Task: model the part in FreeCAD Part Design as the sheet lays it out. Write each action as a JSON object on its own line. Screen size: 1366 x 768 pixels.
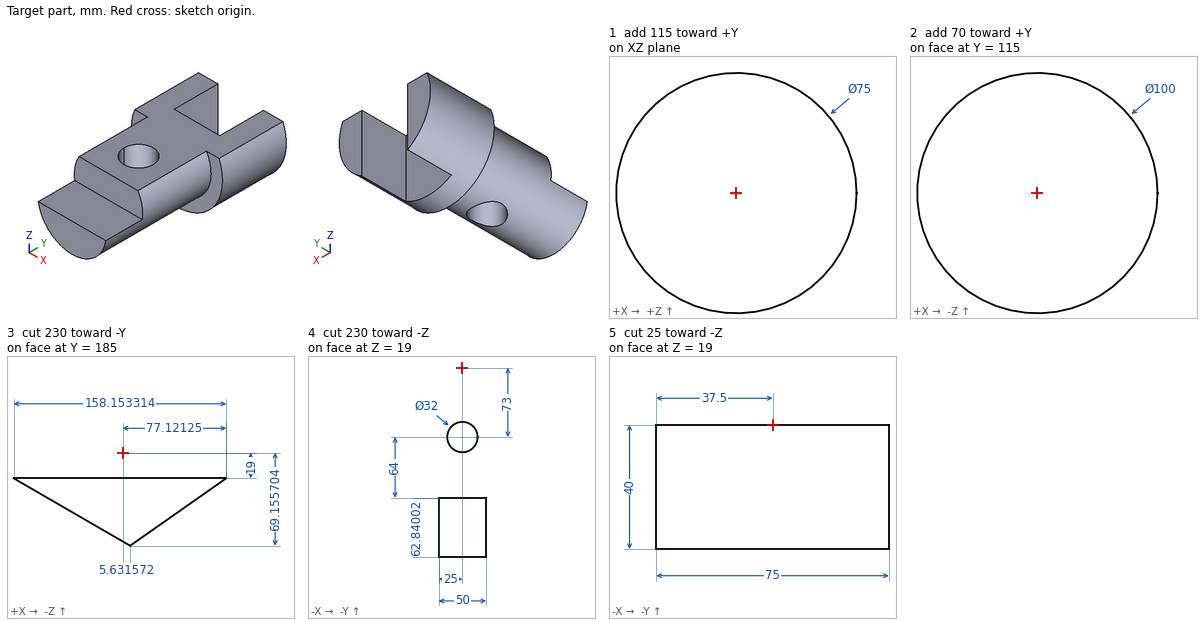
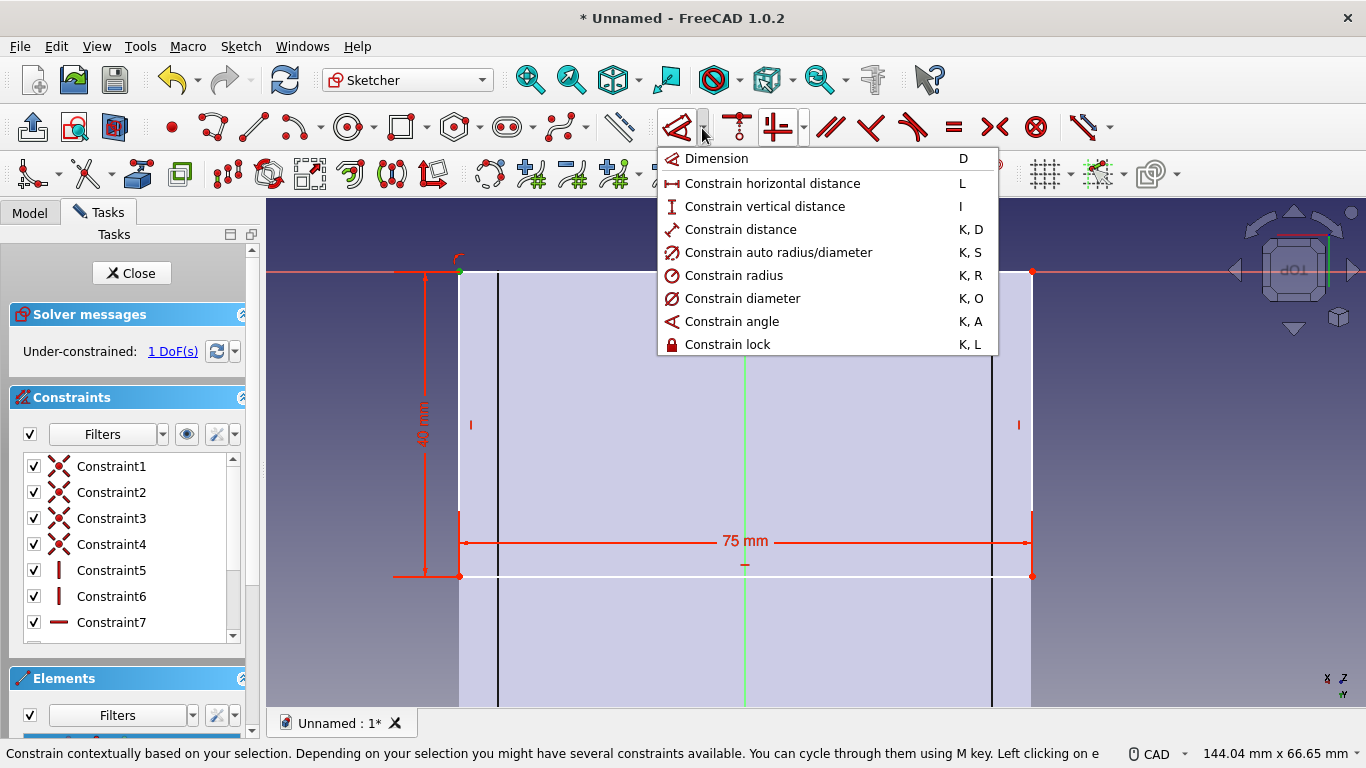
{"action": "left_click", "coordinate": [828, 184]}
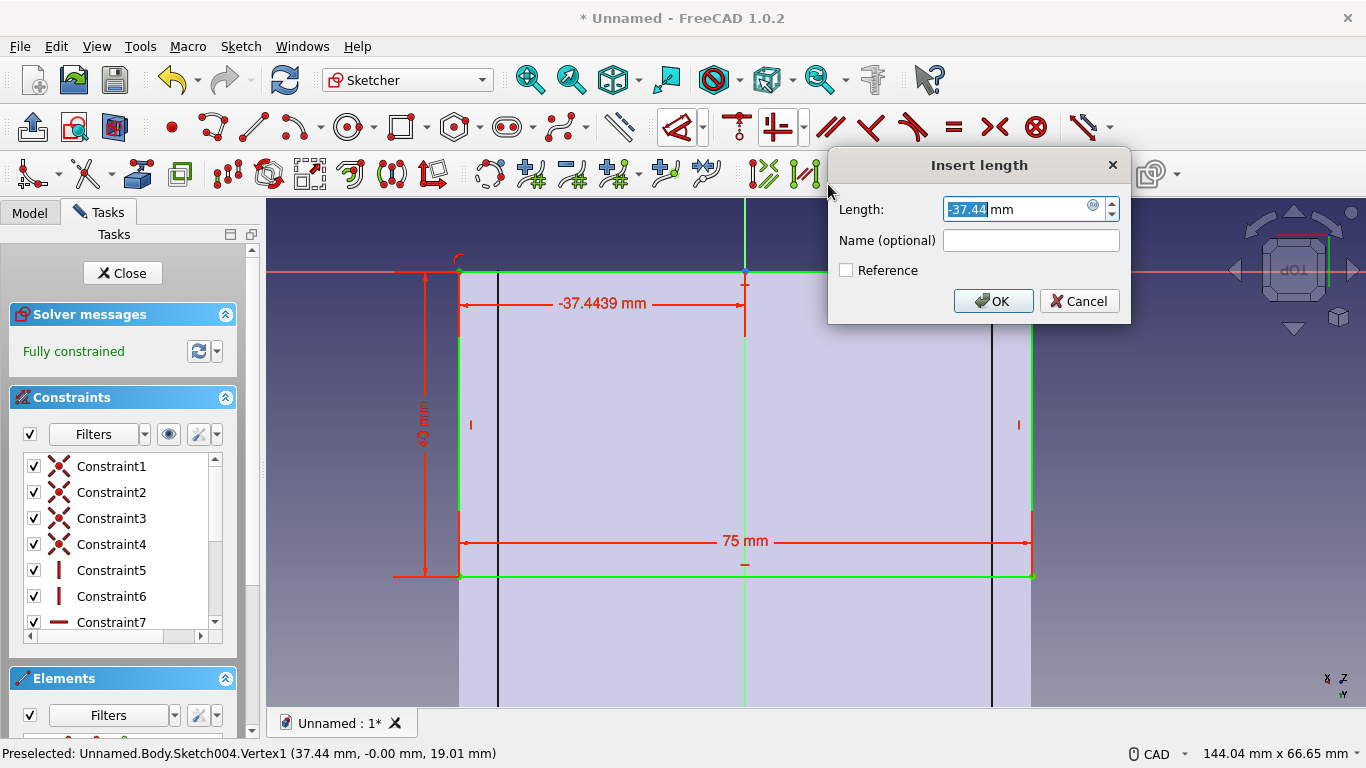
{"action": "type", "text": "-37.5"}
{"action": "key", "text": "Return"}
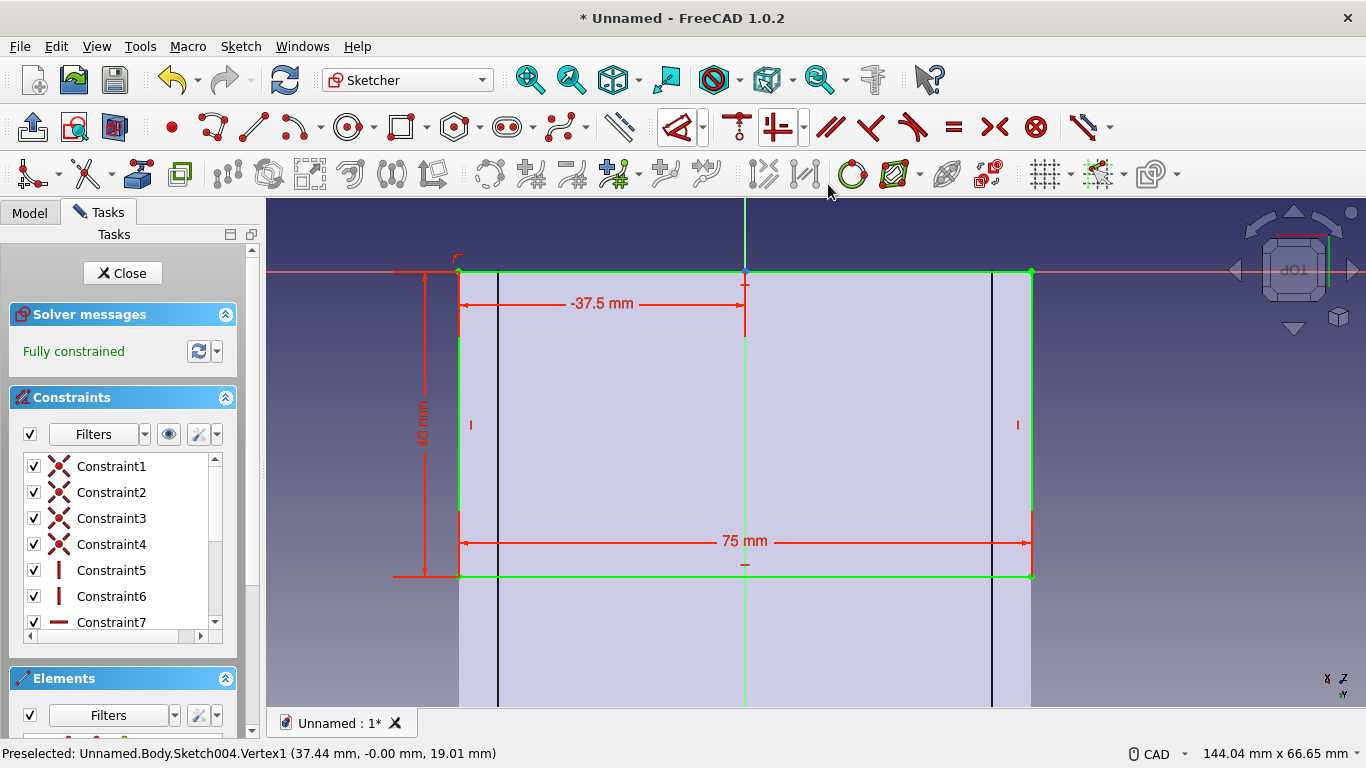
{"action": "left_click", "coordinate": [123, 273]}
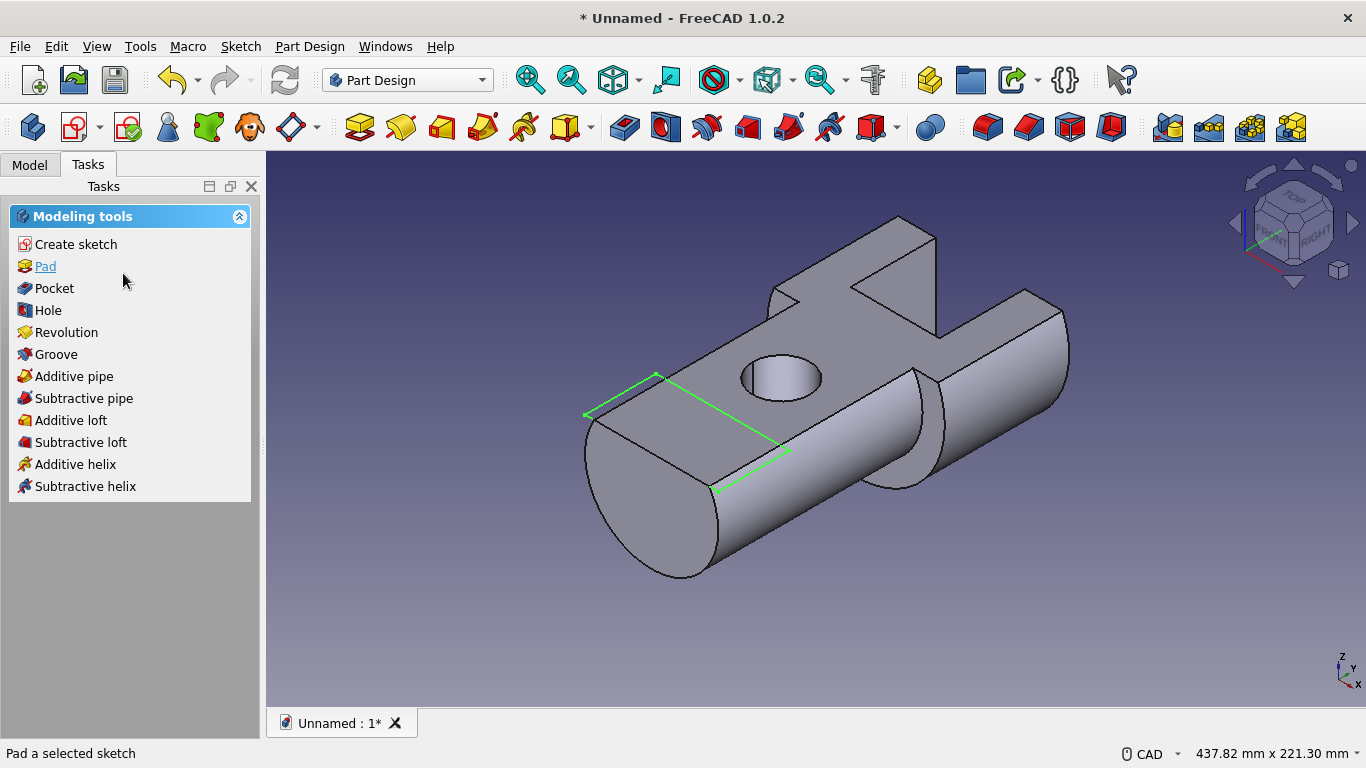
{"action": "left_click", "coordinate": [625, 128]}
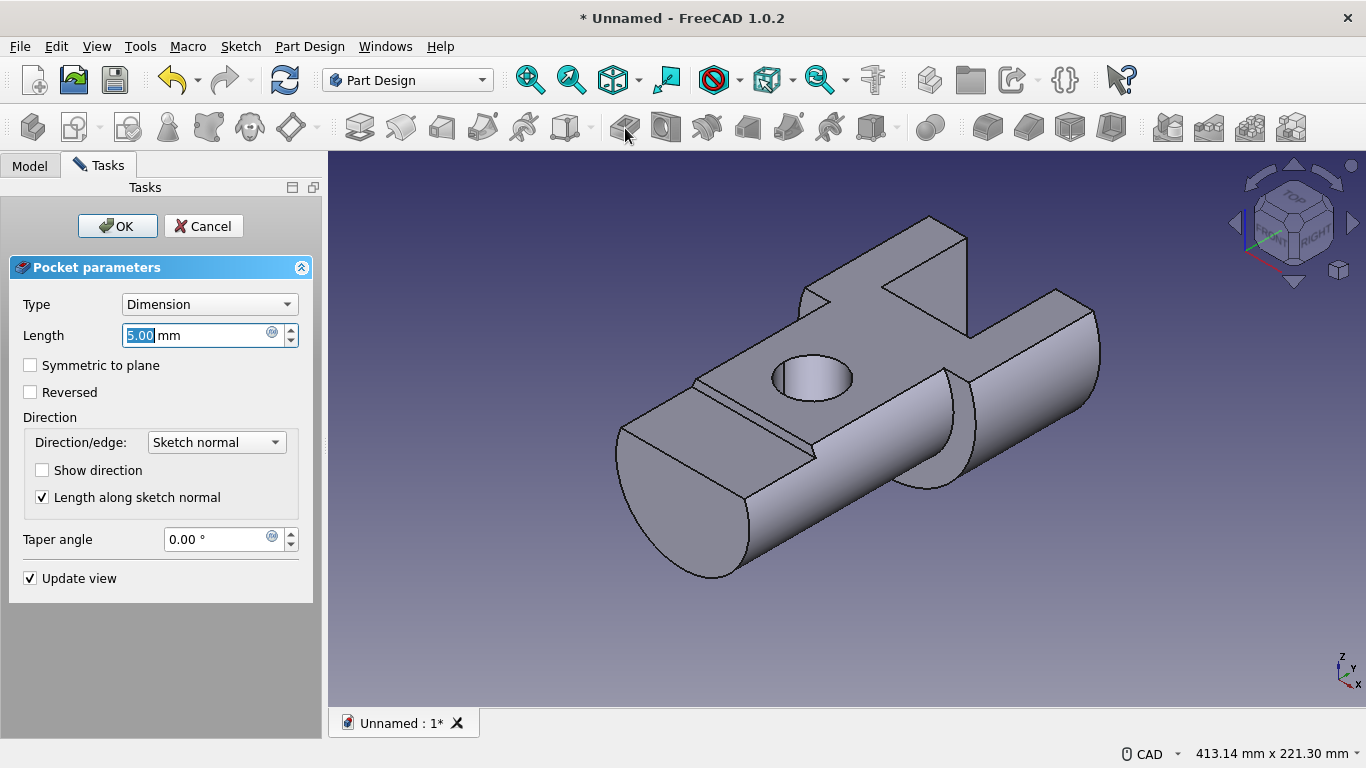
{"action": "type", "text": "25"}
{"action": "key", "text": "Tab"}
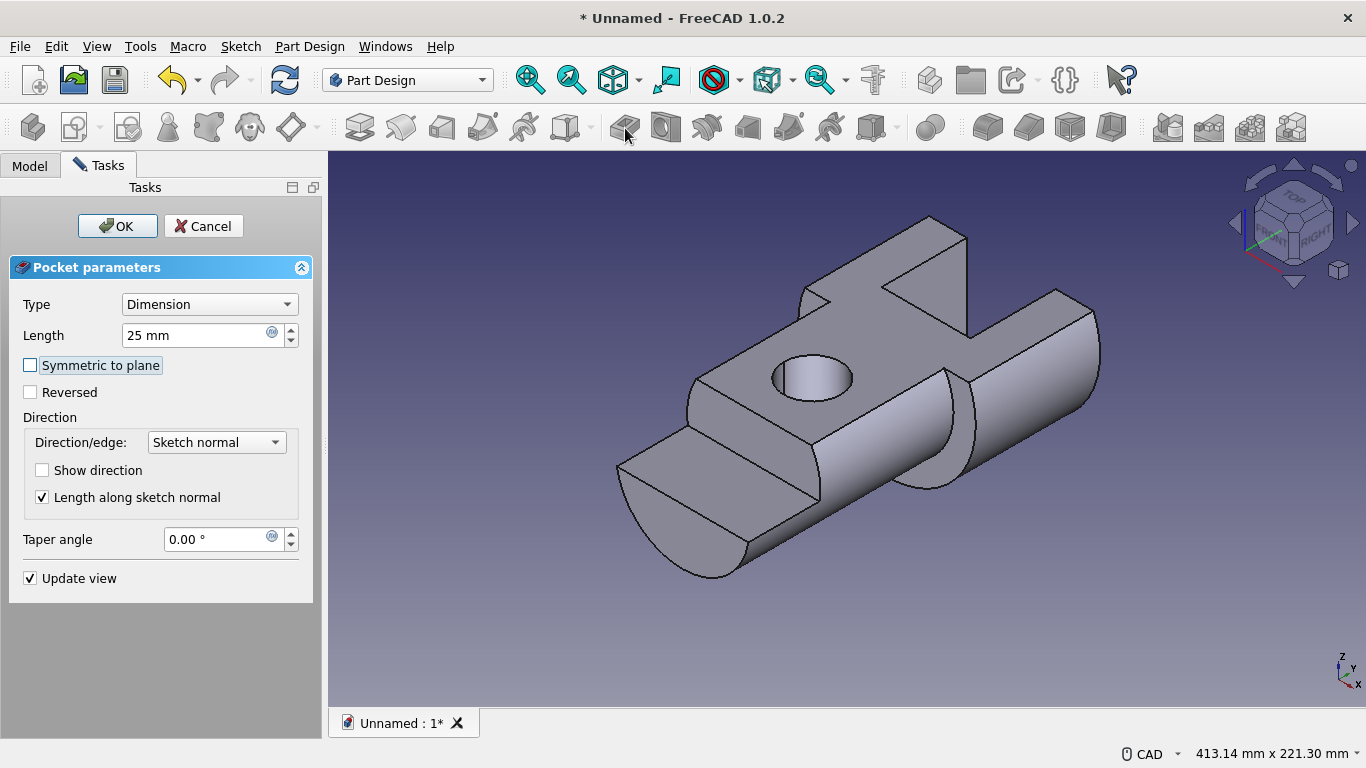
{"action": "left_click", "coordinate": [118, 226]}